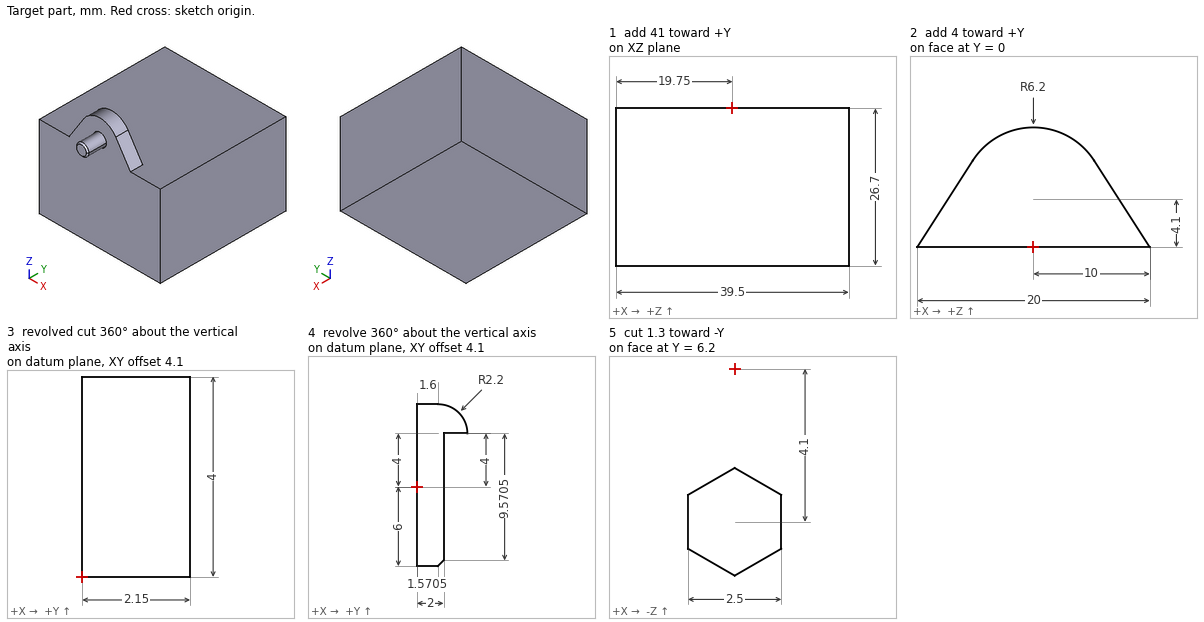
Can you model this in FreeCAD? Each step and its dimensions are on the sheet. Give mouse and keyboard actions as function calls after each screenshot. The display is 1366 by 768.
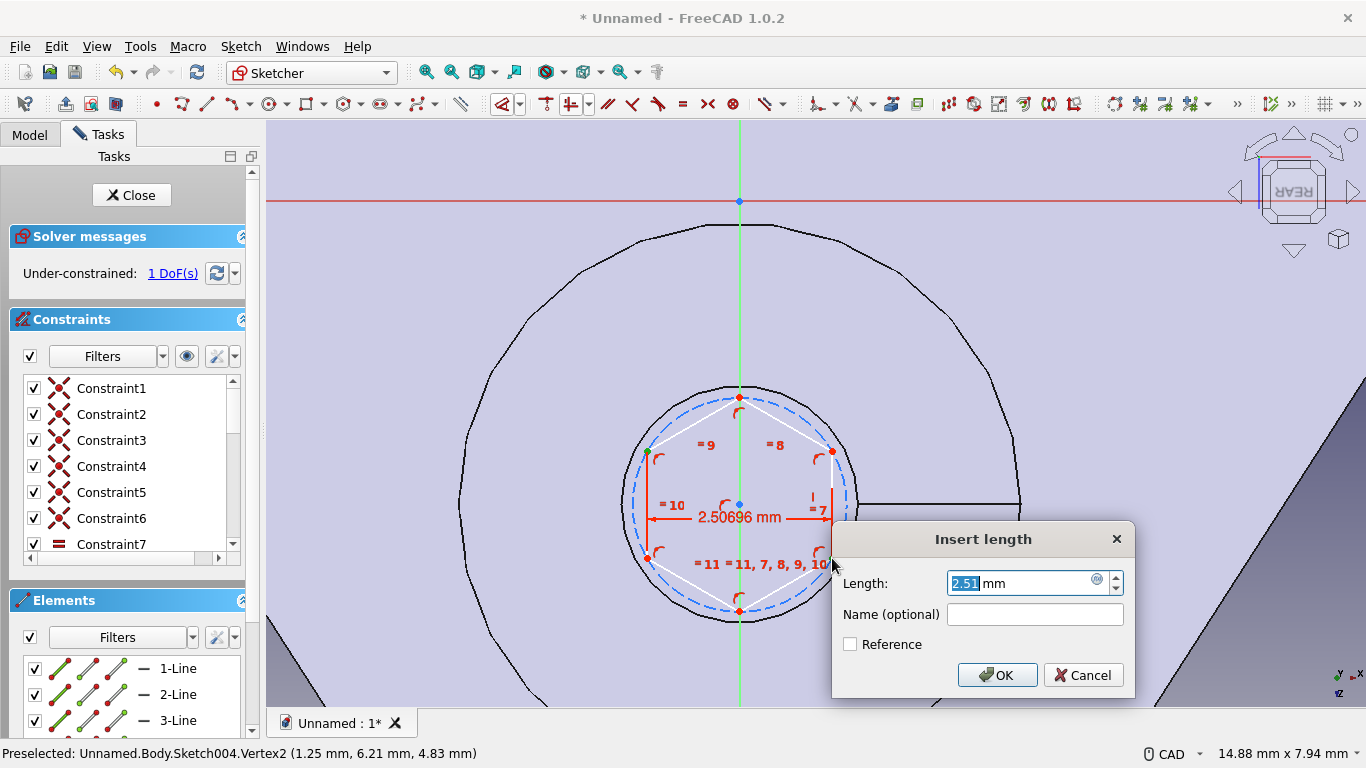
text(2.5)
key(Return)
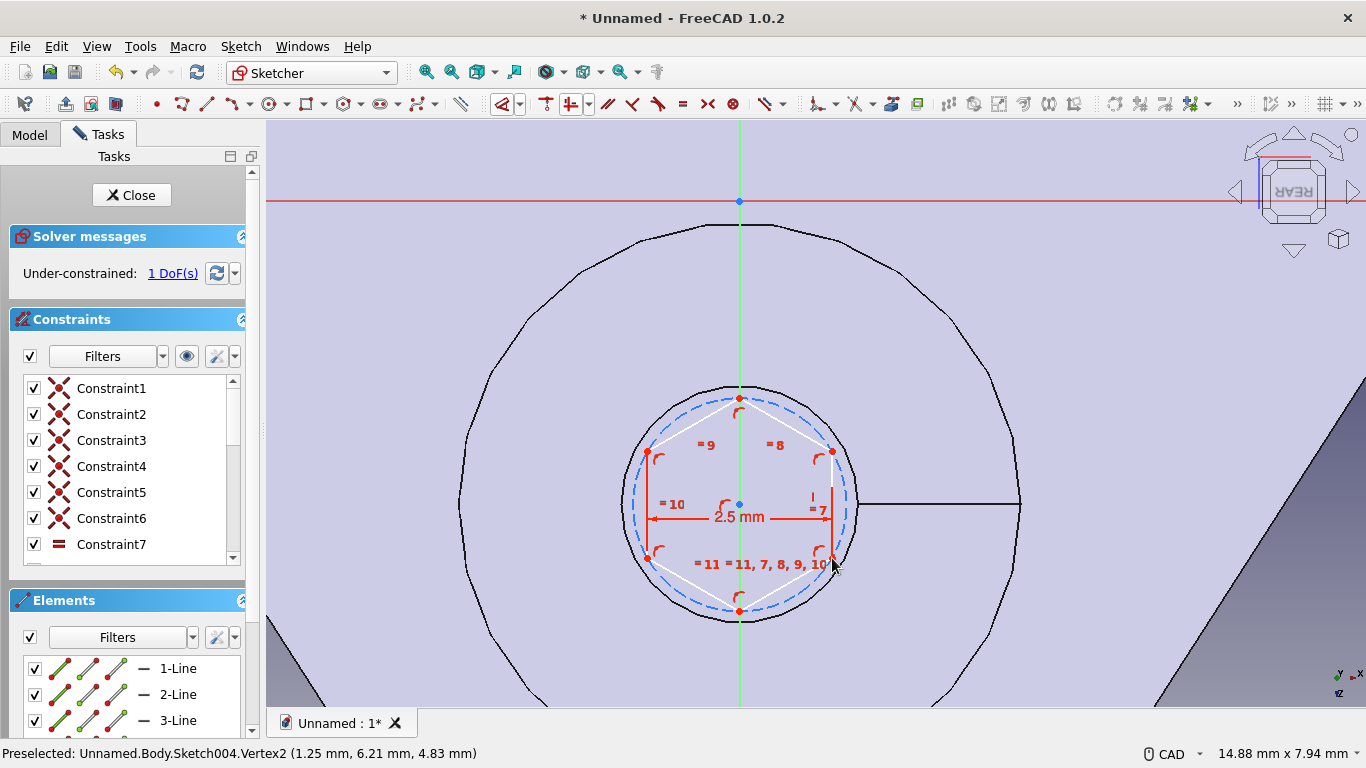
click(740, 505)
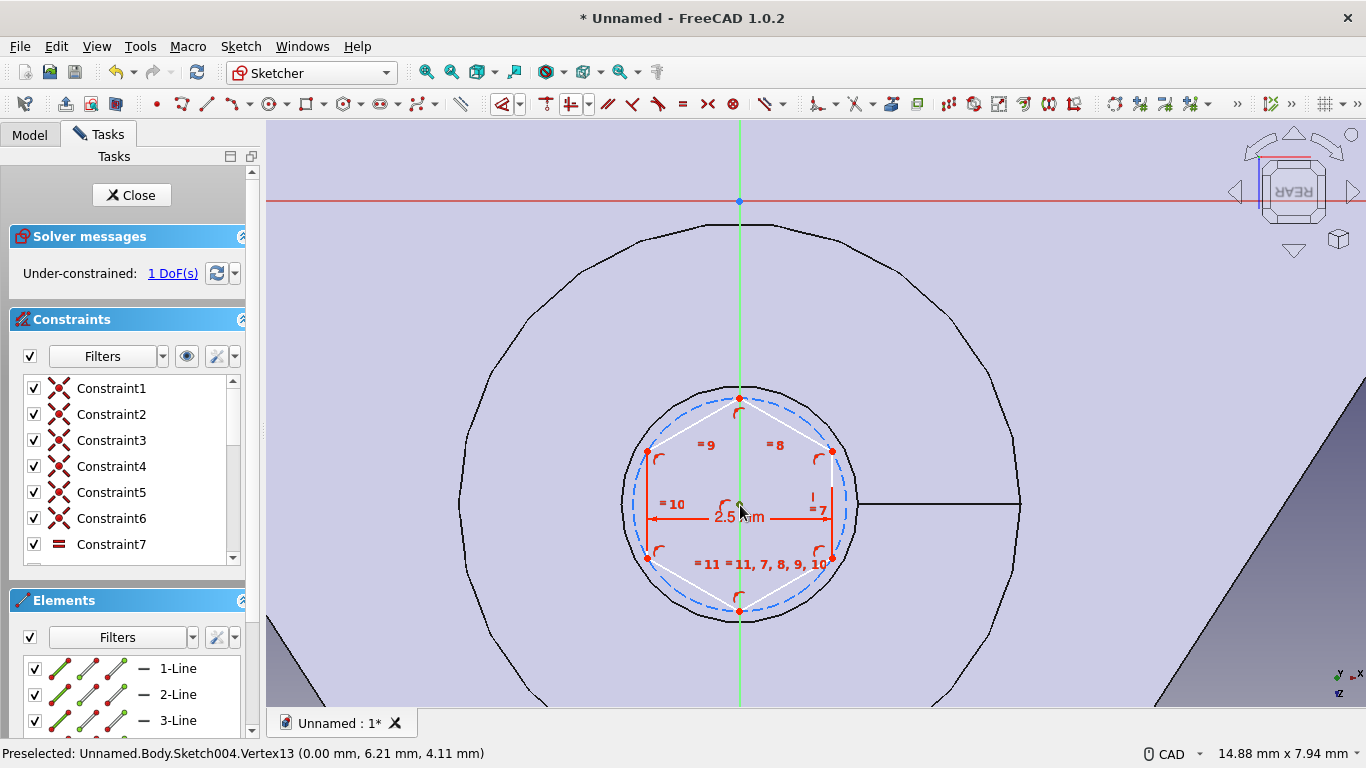
key(i)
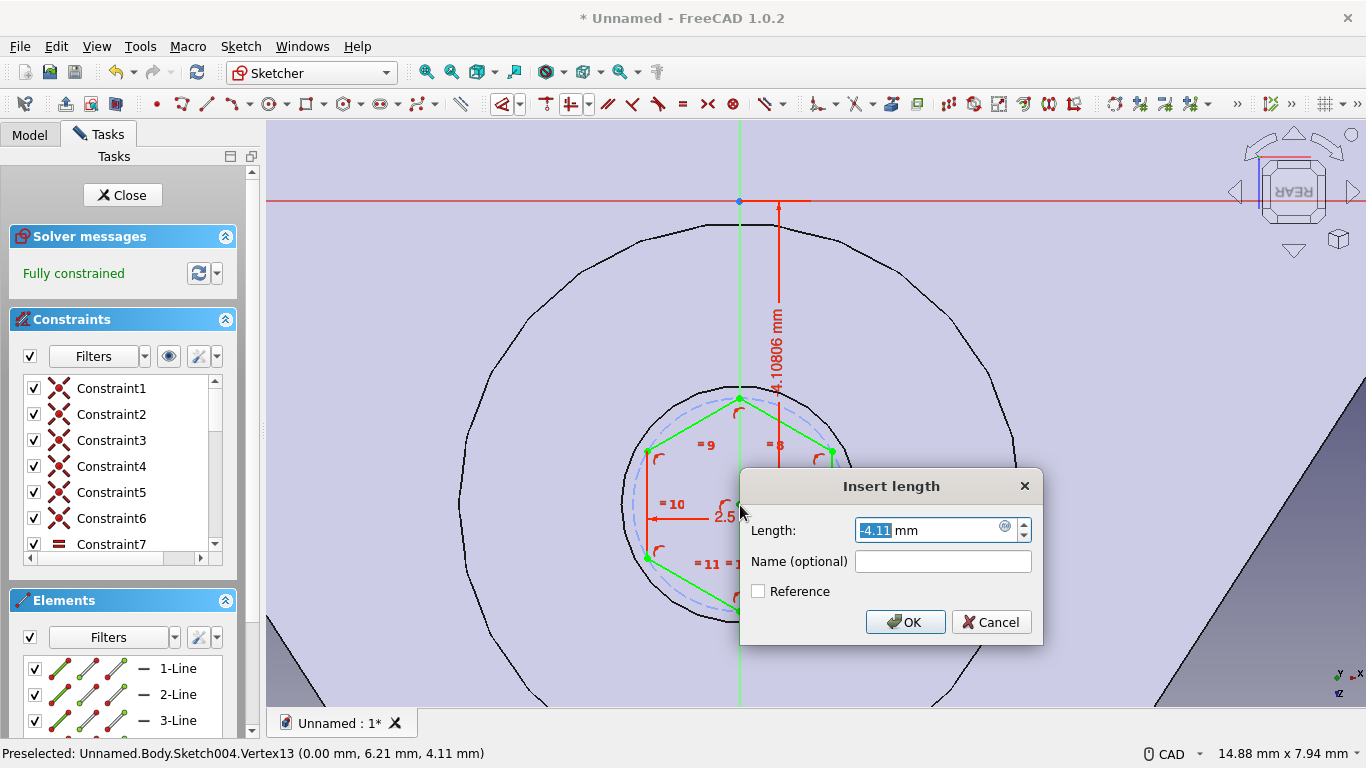
text(-4.1)
key(Return)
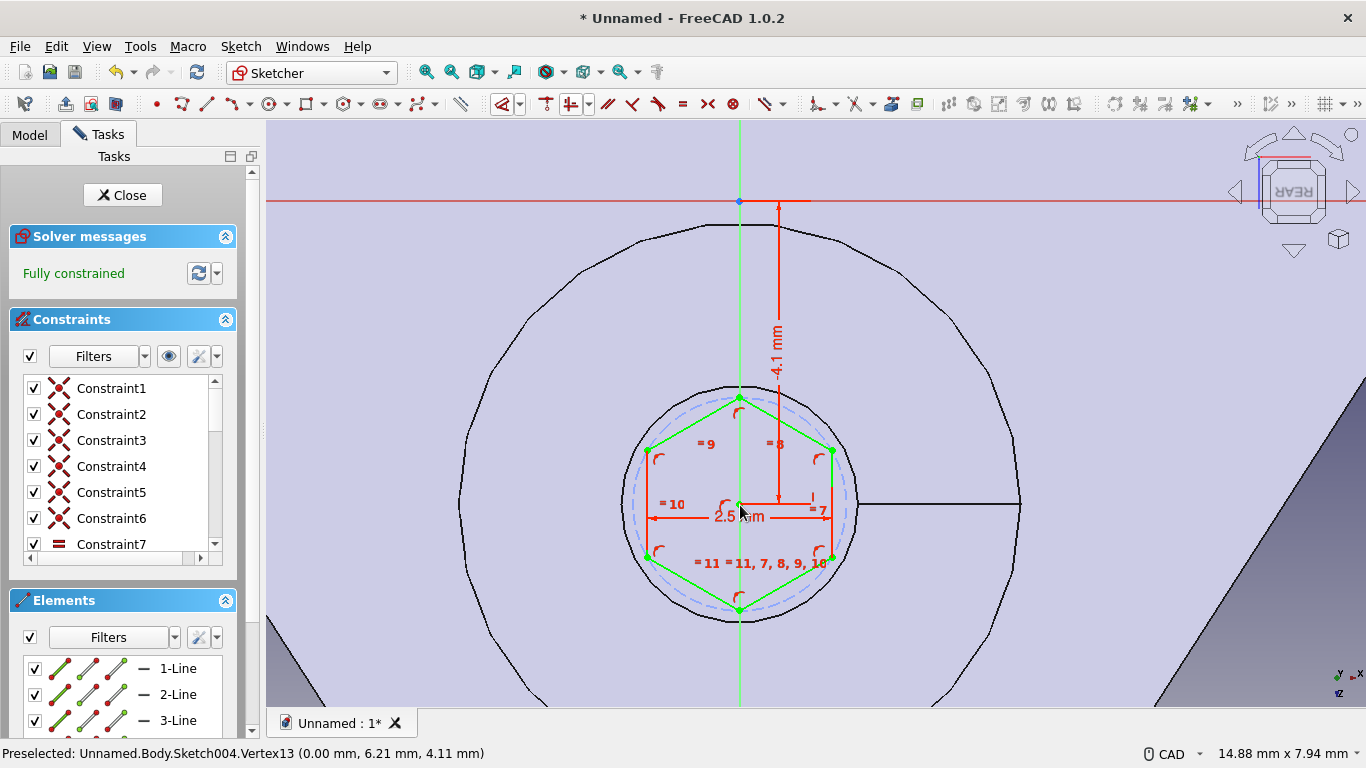
click(123, 195)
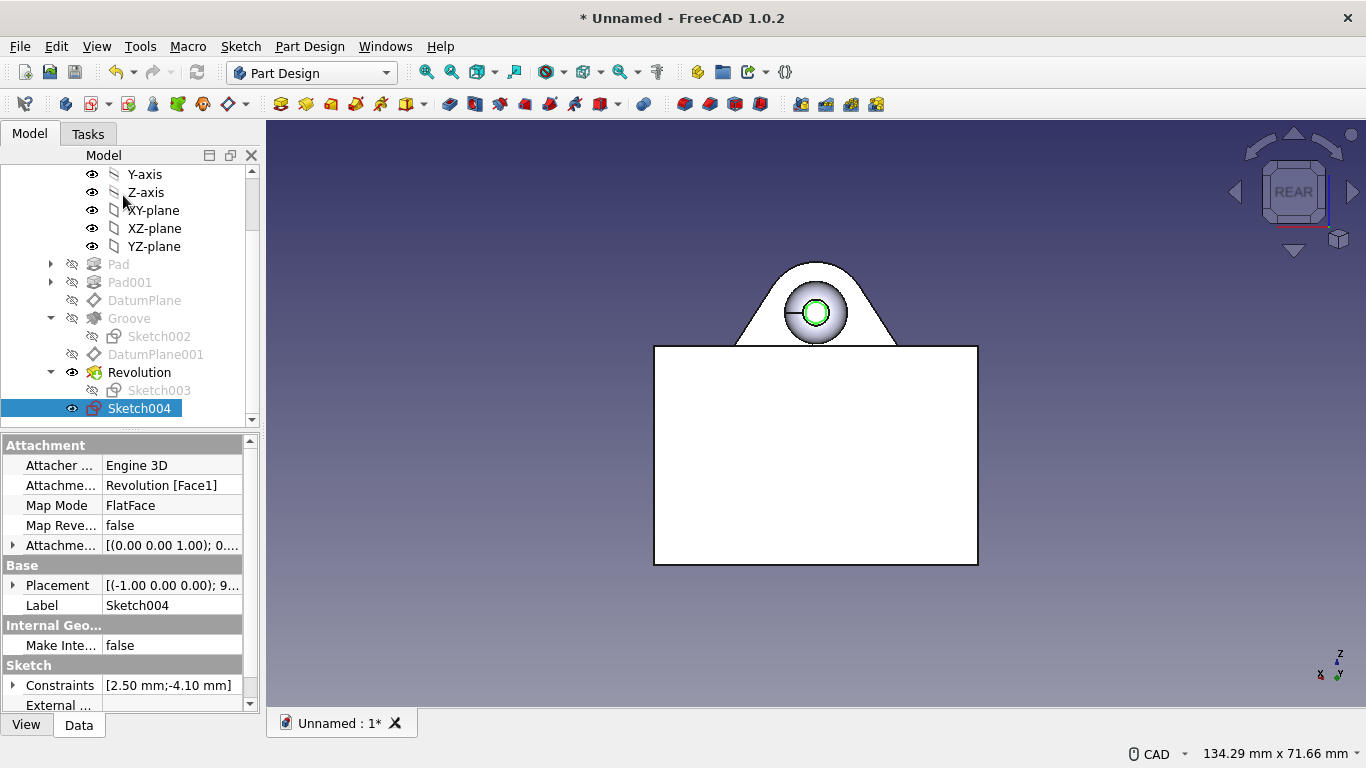
click(450, 104)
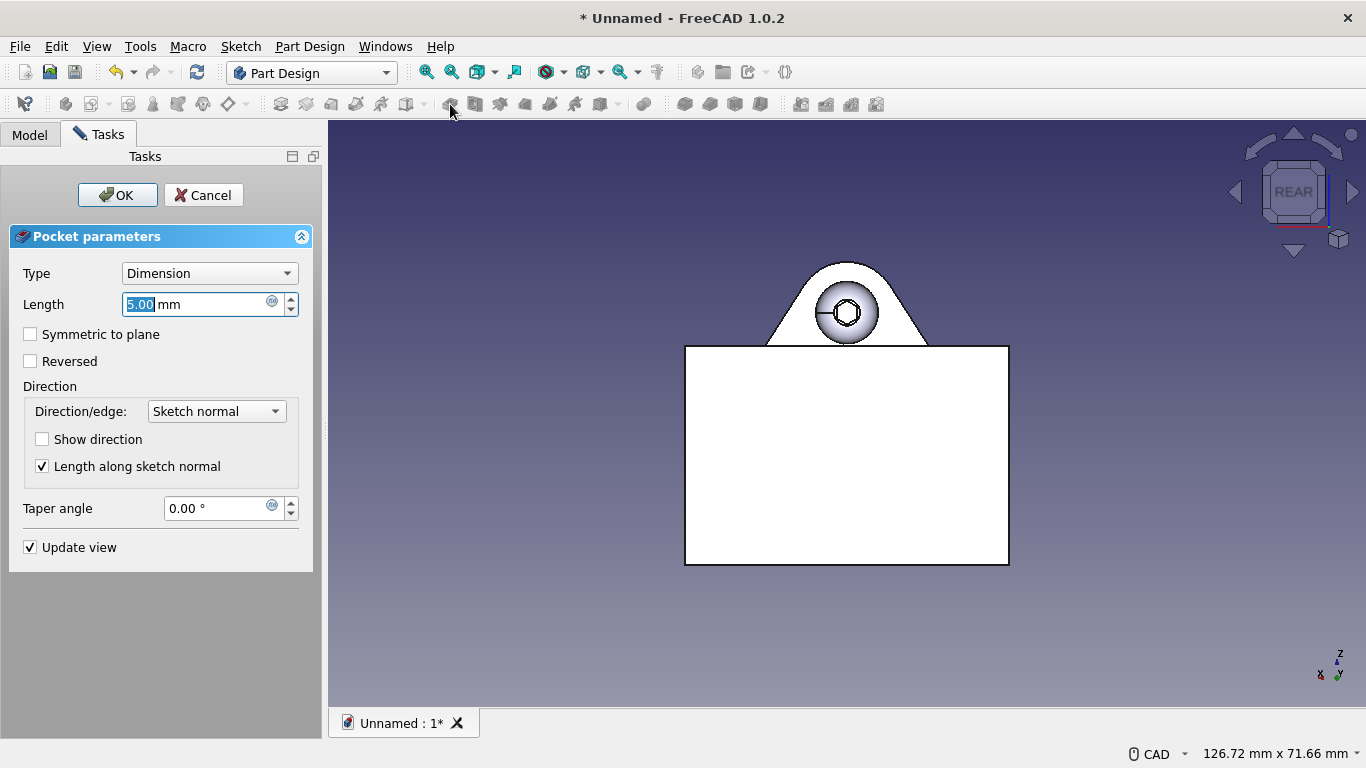
text(1.3)
key(Tab)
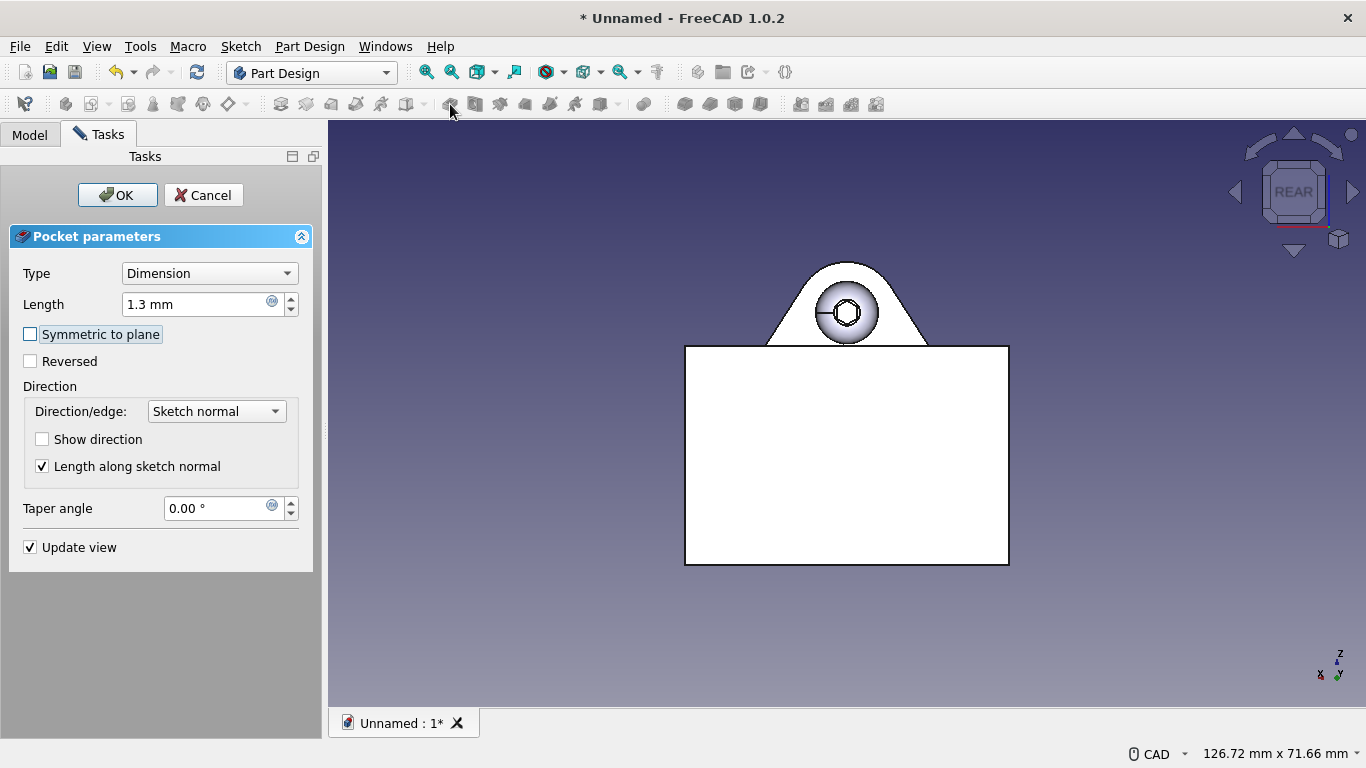
click(118, 195)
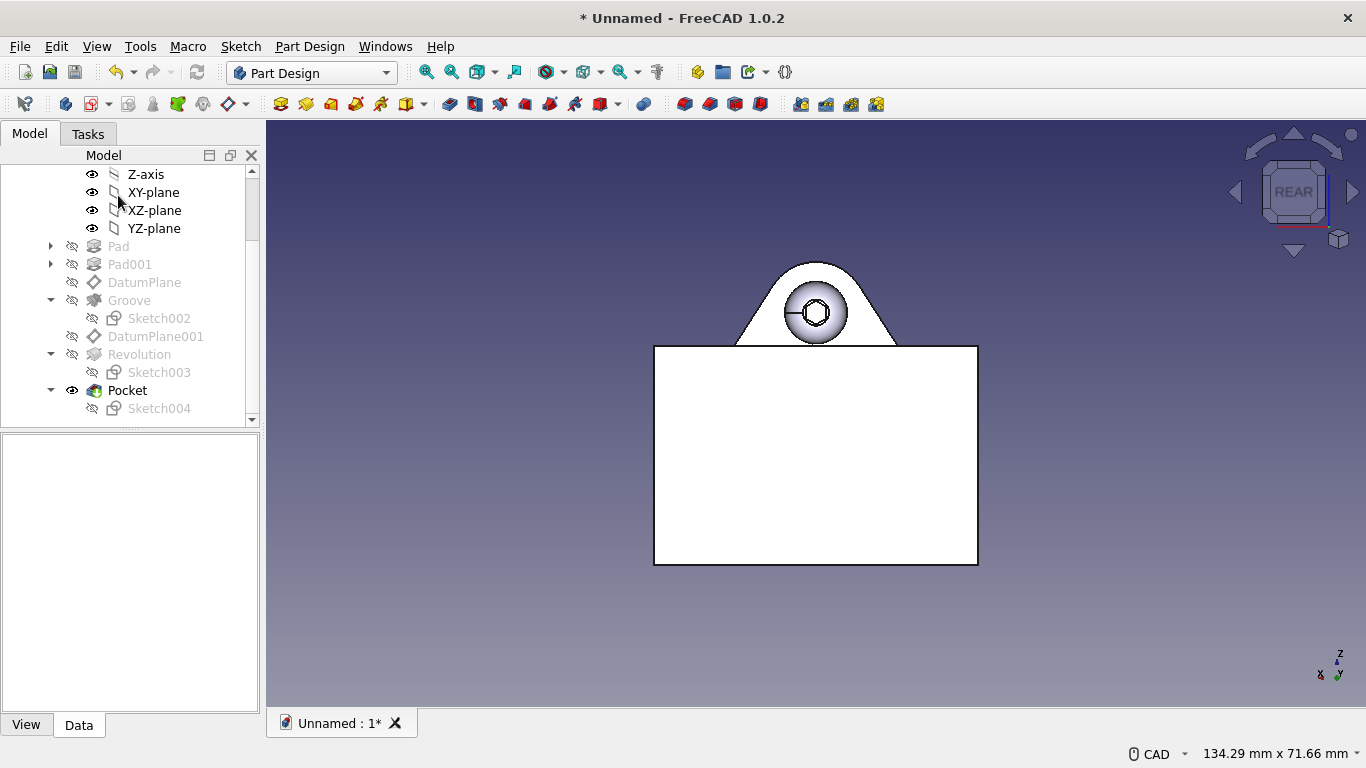
key(0)